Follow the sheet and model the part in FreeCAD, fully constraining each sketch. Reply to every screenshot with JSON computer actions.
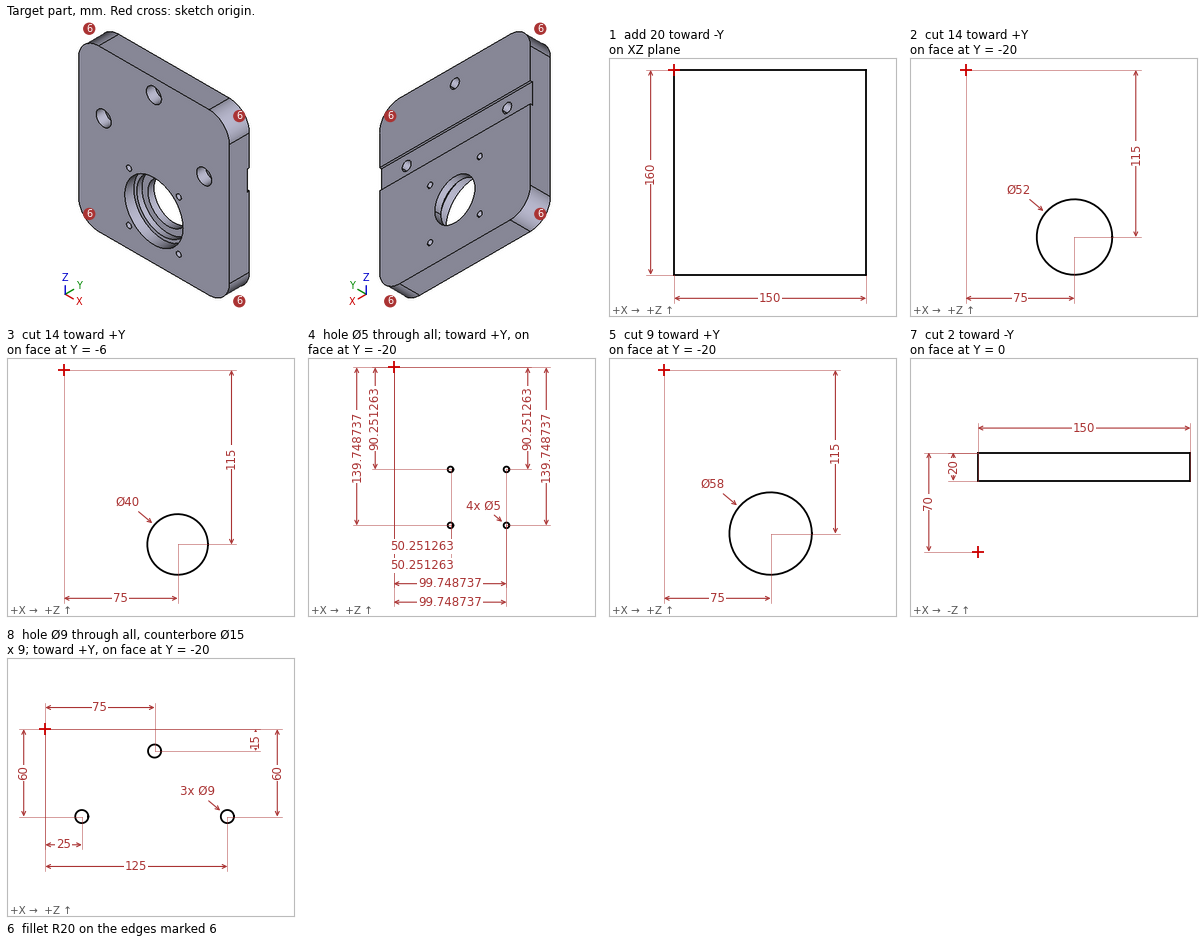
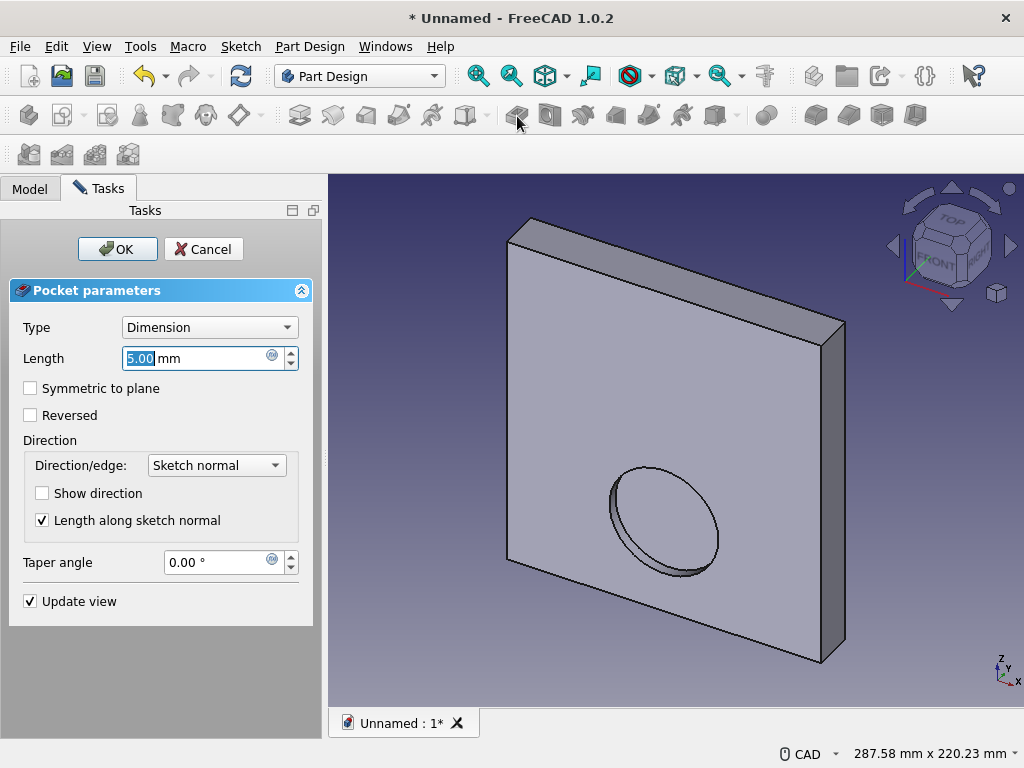
{"action": "type", "text": "14"}
{"action": "key", "text": "Tab"}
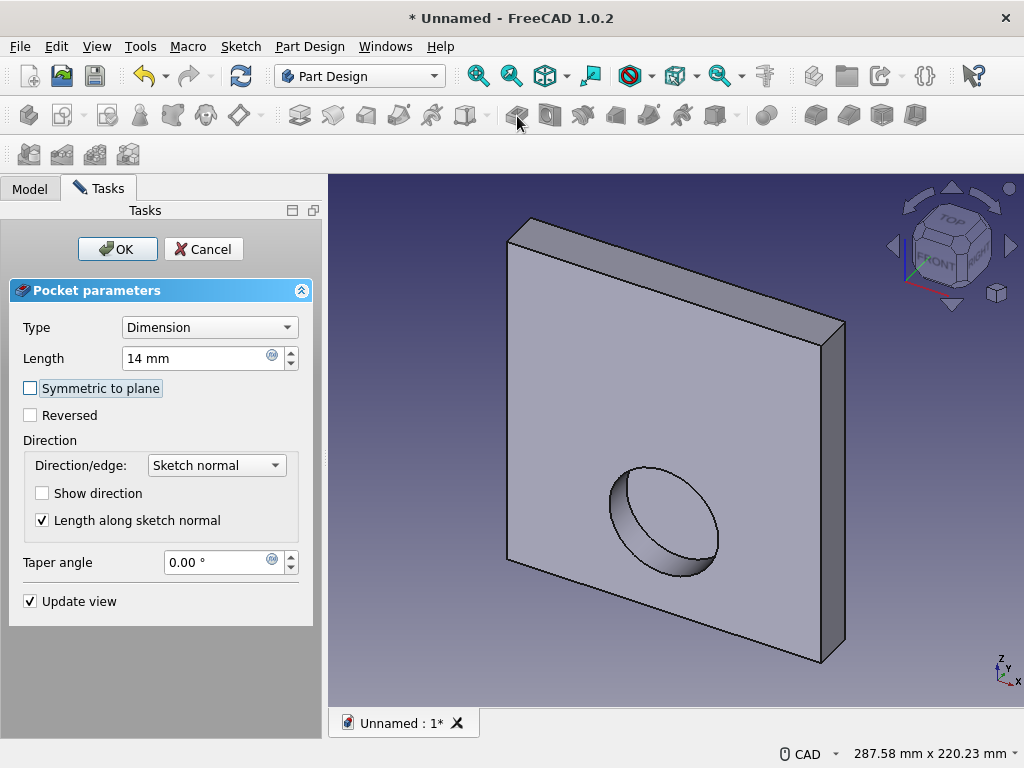
{"action": "left_click", "coordinate": [118, 249]}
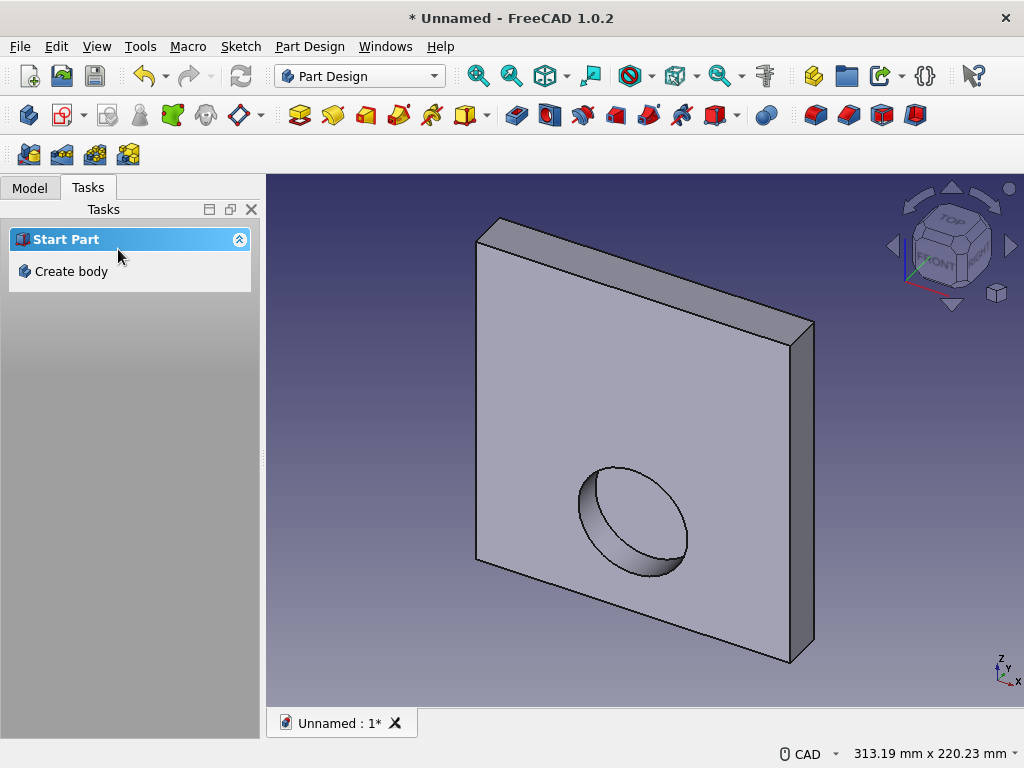
{"action": "left_click", "coordinate": [650, 504]}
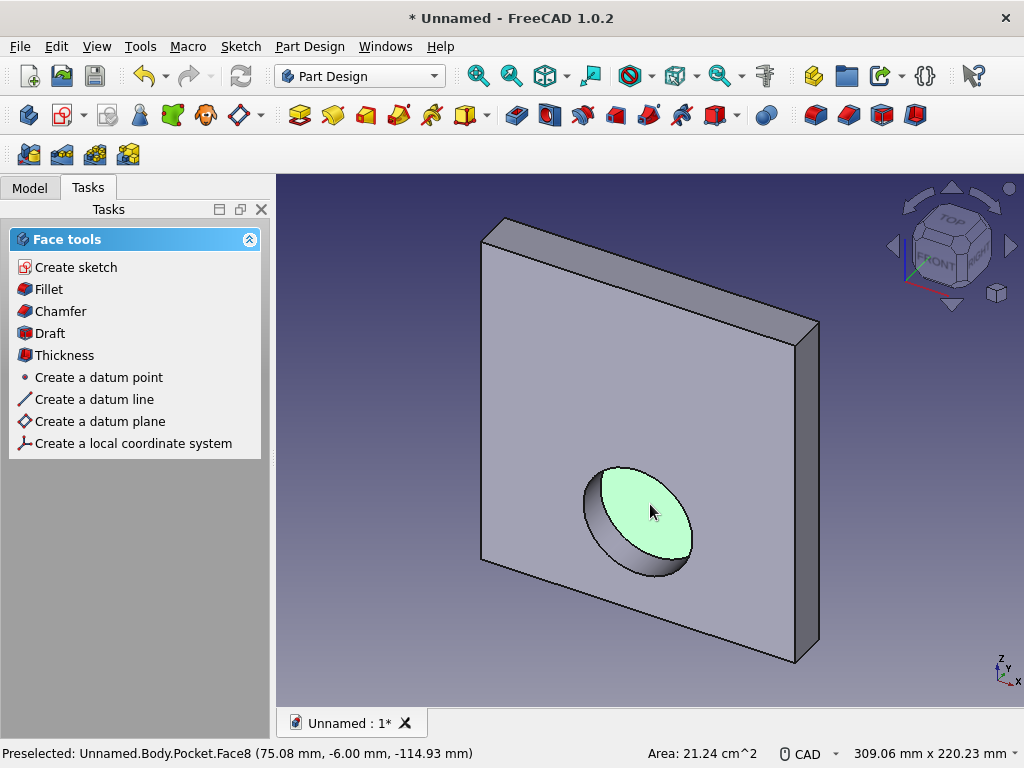
{"action": "left_click", "coordinate": [62, 116]}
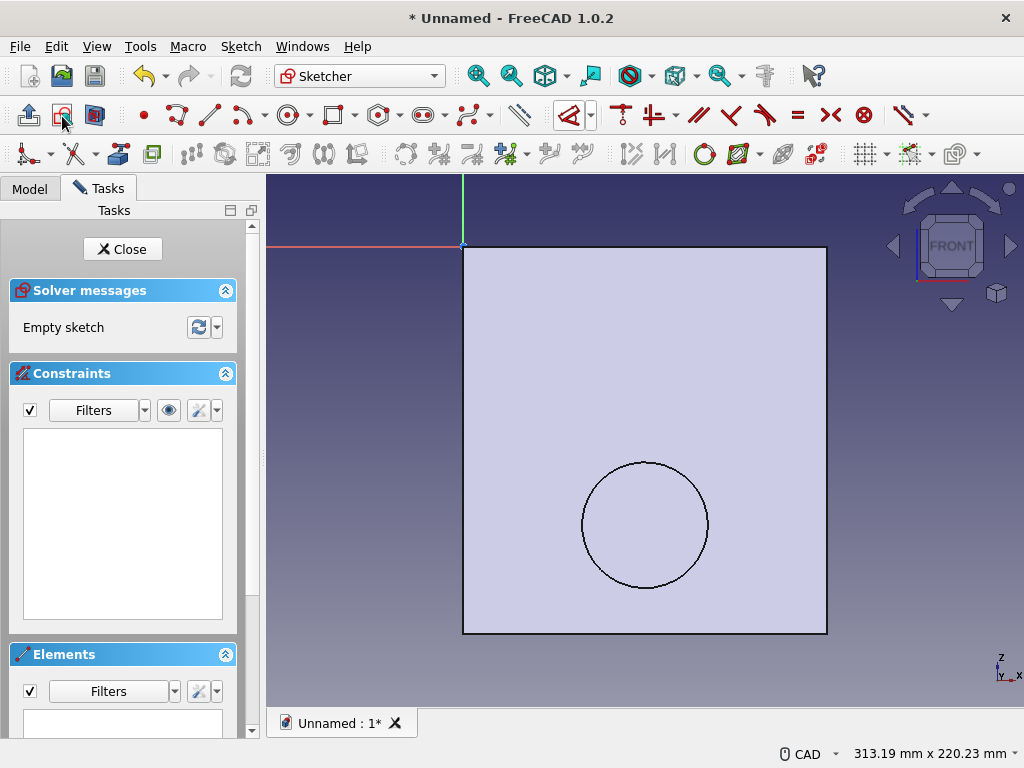
{"action": "scroll", "coordinate": [675, 562], "scroll_direction": "up", "scroll_amount": 6}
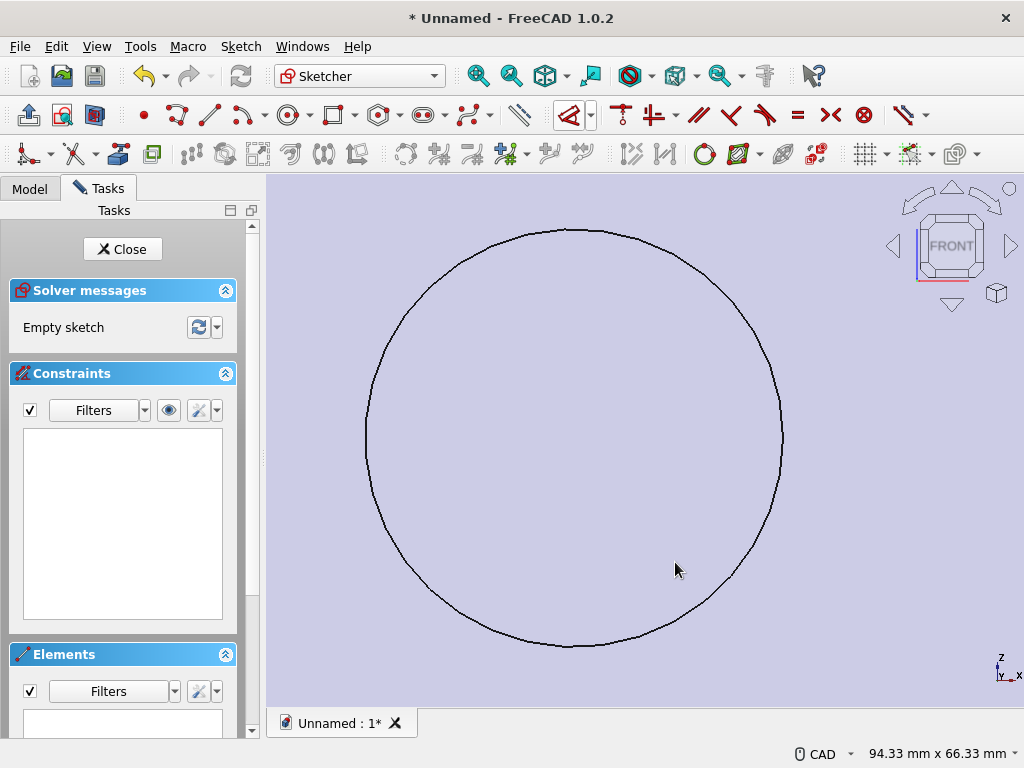
{"action": "left_click", "coordinate": [288, 116]}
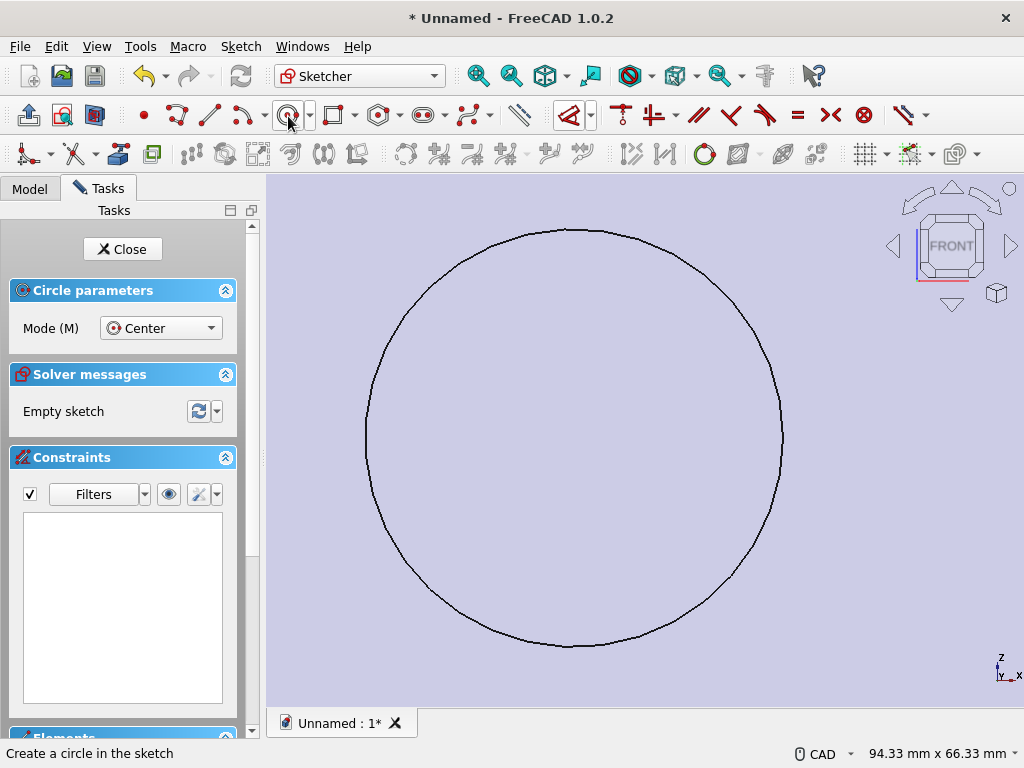
{"action": "left_click", "coordinate": [574, 438]}
{"action": "left_click", "coordinate": [688, 325]}
{"action": "key", "text": "Escape"}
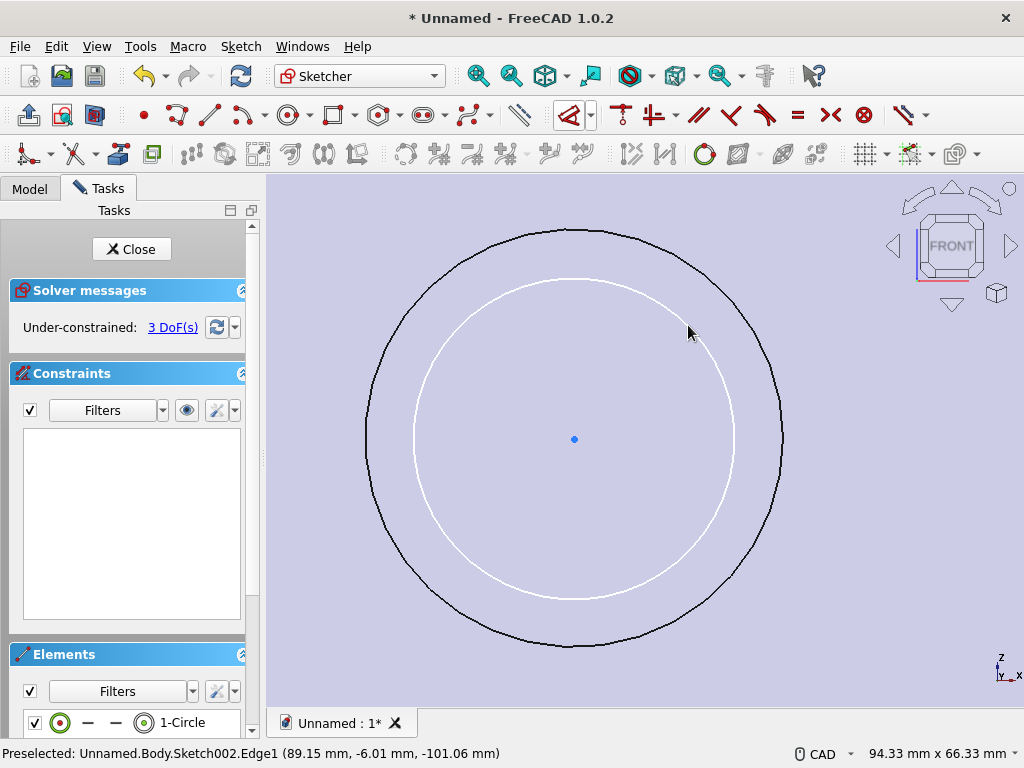
{"action": "left_click", "coordinate": [687, 325]}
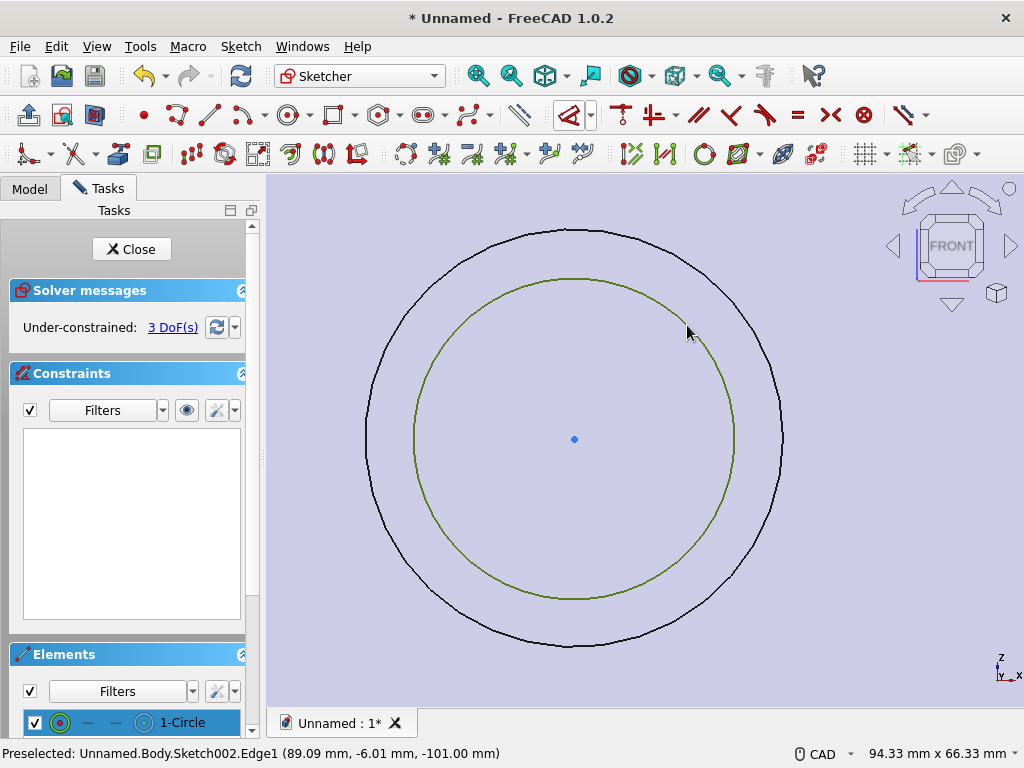
{"action": "key", "text": "k o"}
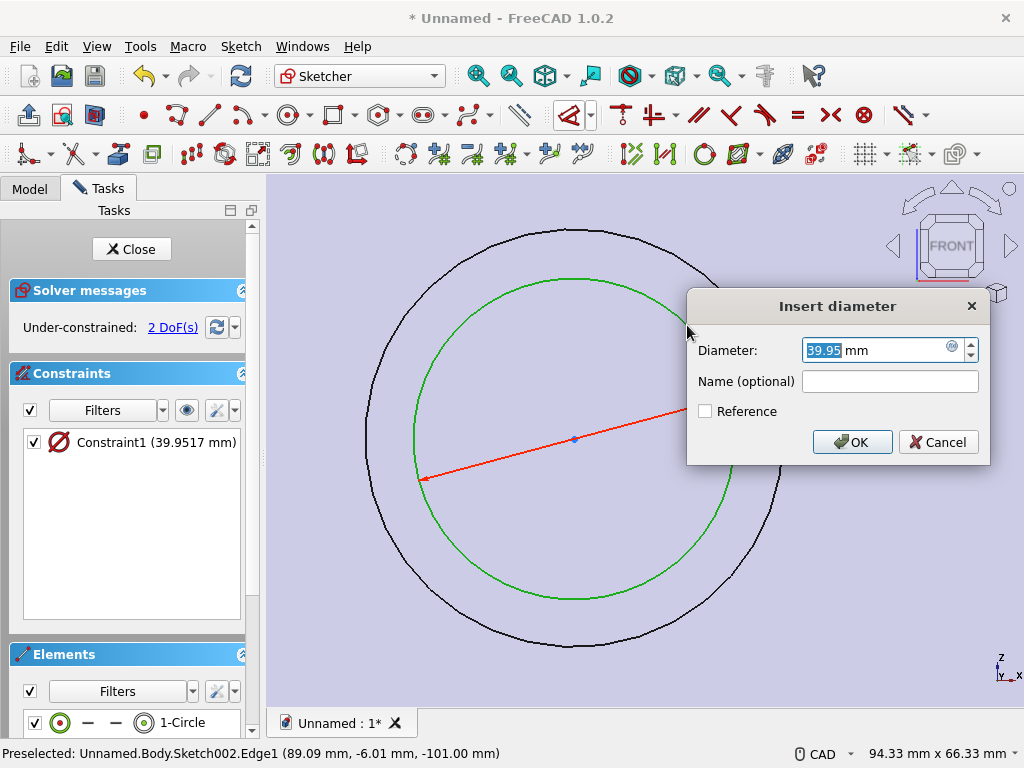
{"action": "type", "text": "40"}
{"action": "key", "text": "Return"}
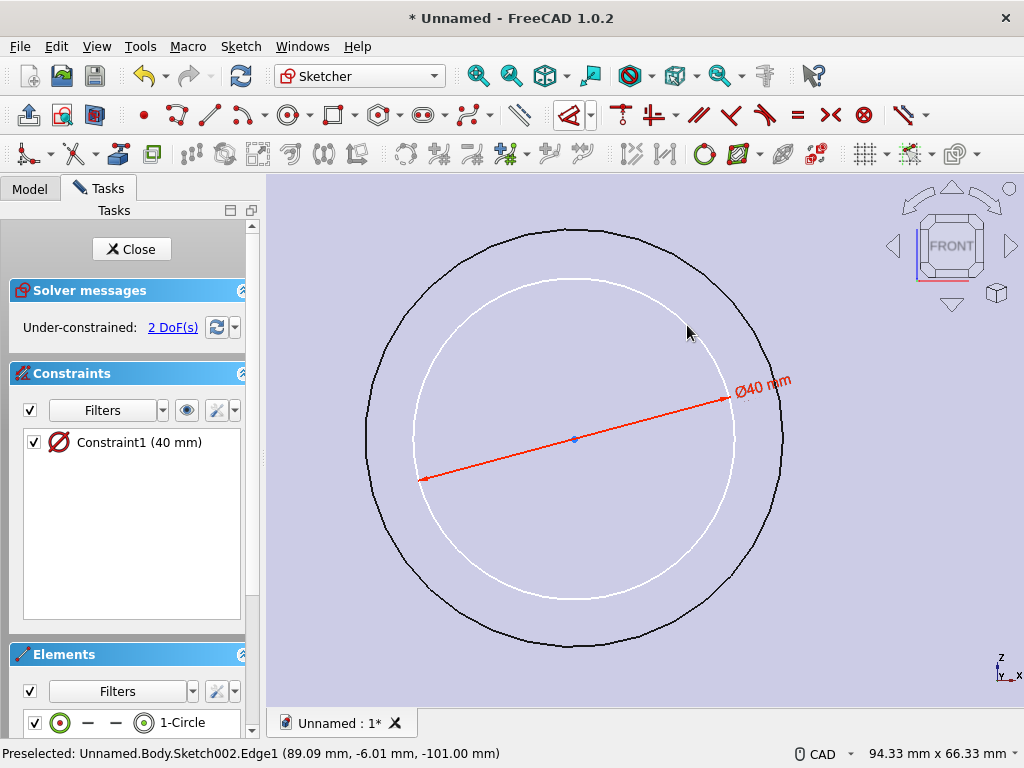
{"action": "left_click", "coordinate": [574, 439]}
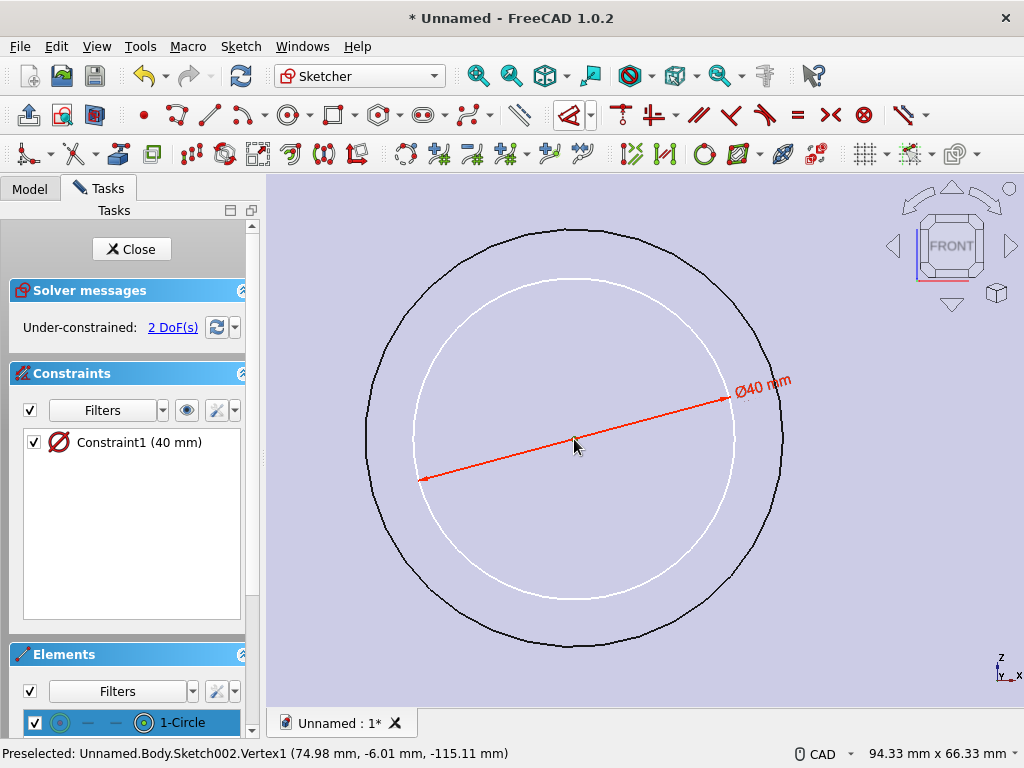
{"action": "left_click", "coordinate": [590, 116]}